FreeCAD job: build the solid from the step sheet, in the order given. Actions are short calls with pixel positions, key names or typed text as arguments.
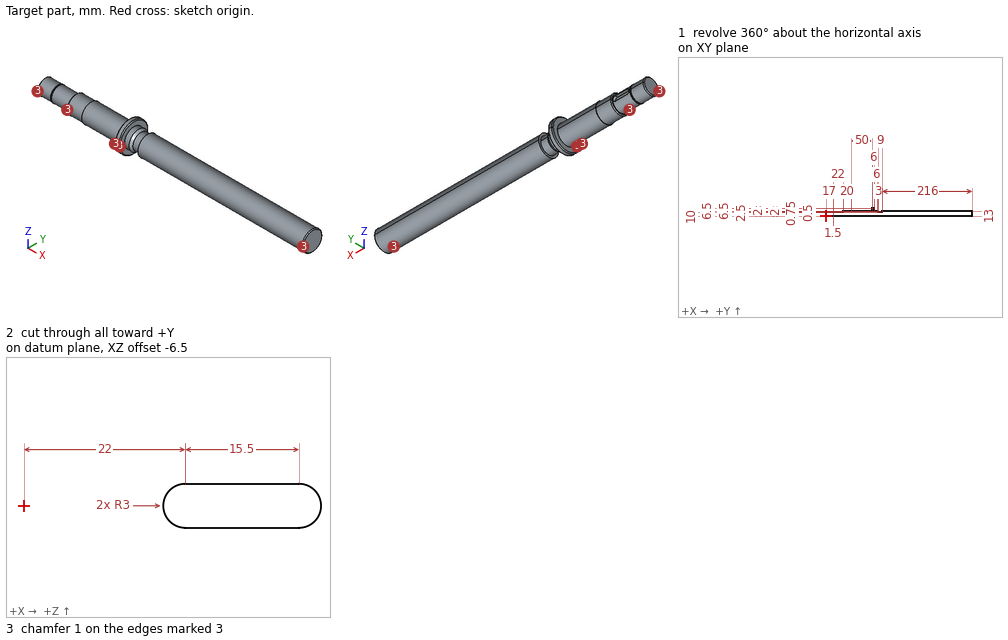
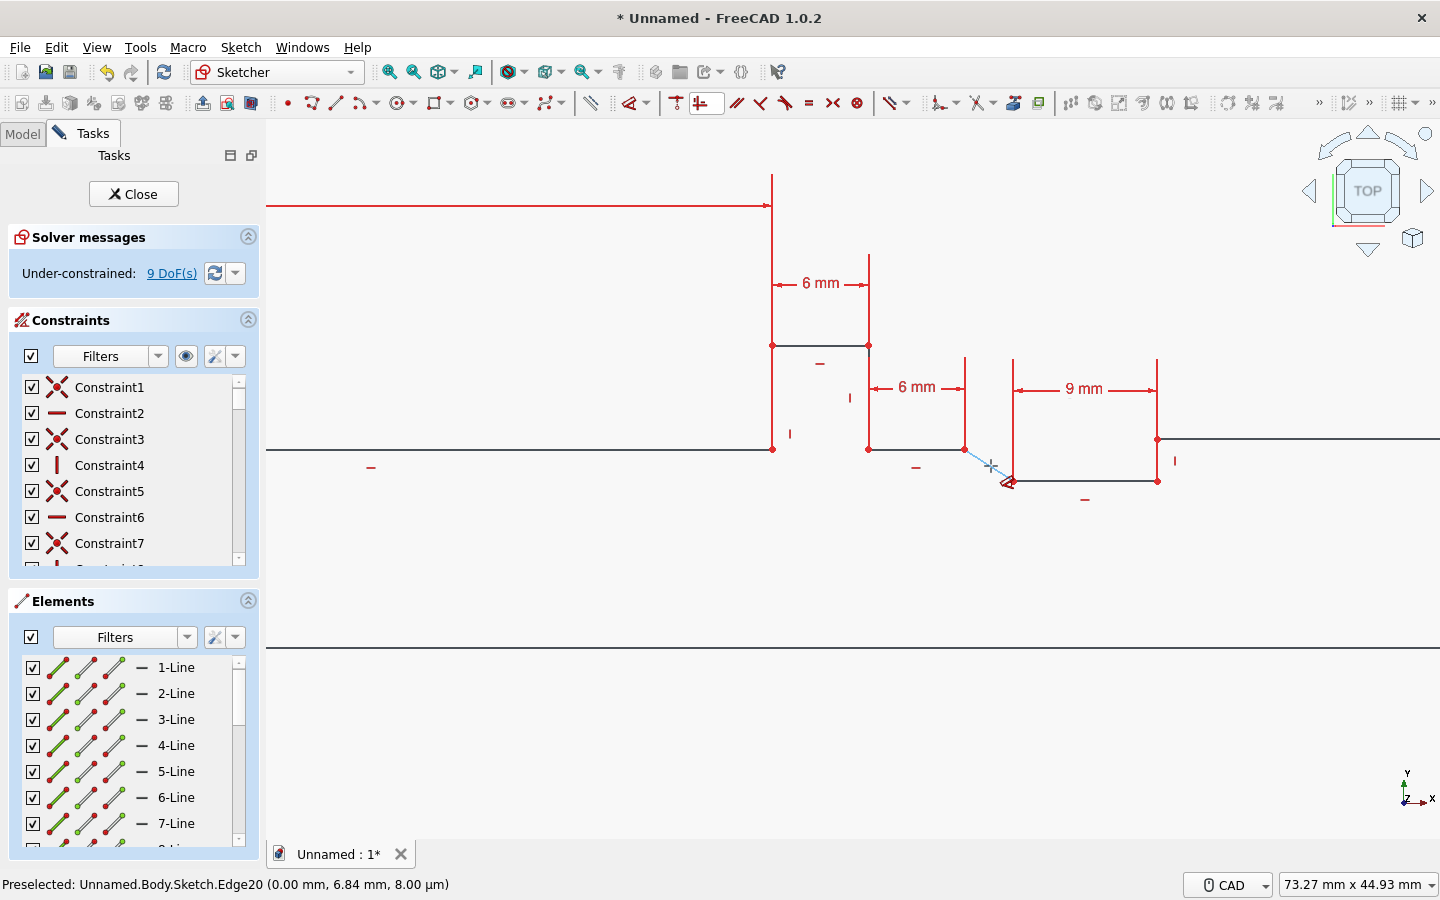
click(989, 465)
click(989, 416)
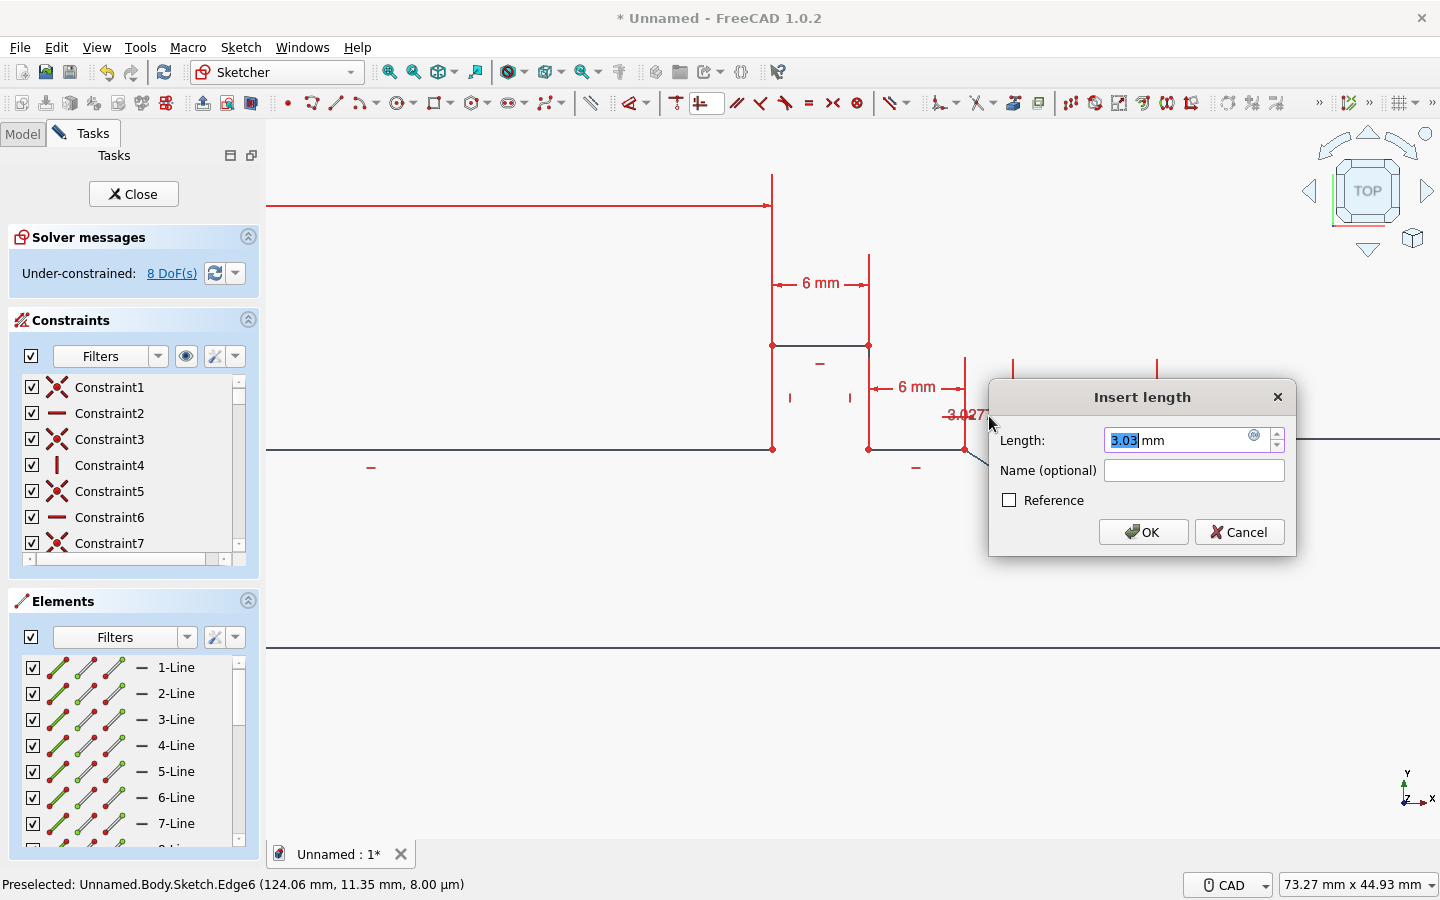
text(3)
key(Return)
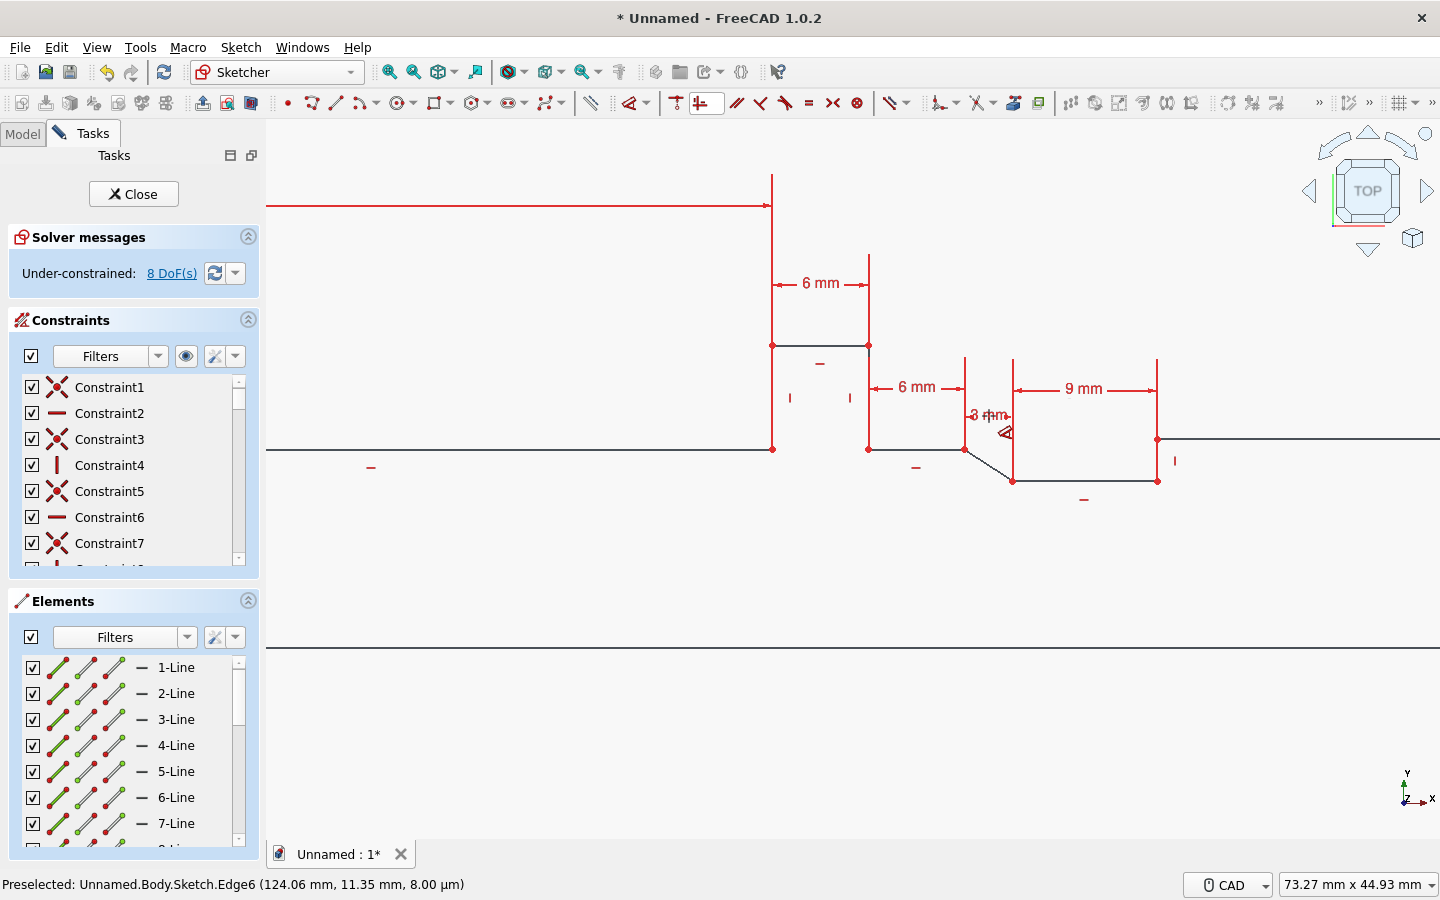
scroll(998, 472, up, 2)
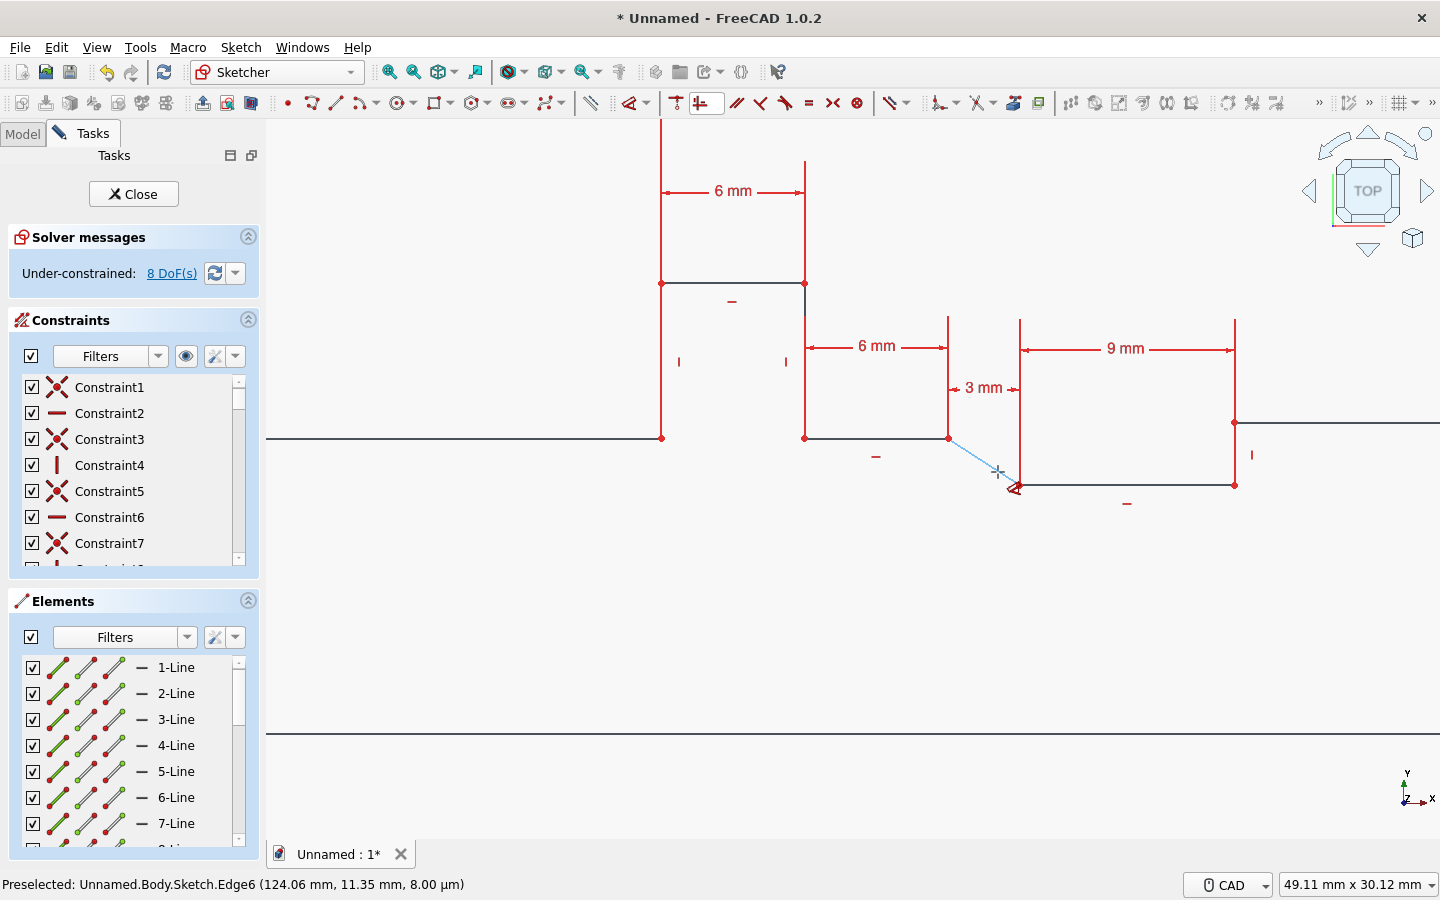
click(998, 471)
click(914, 462)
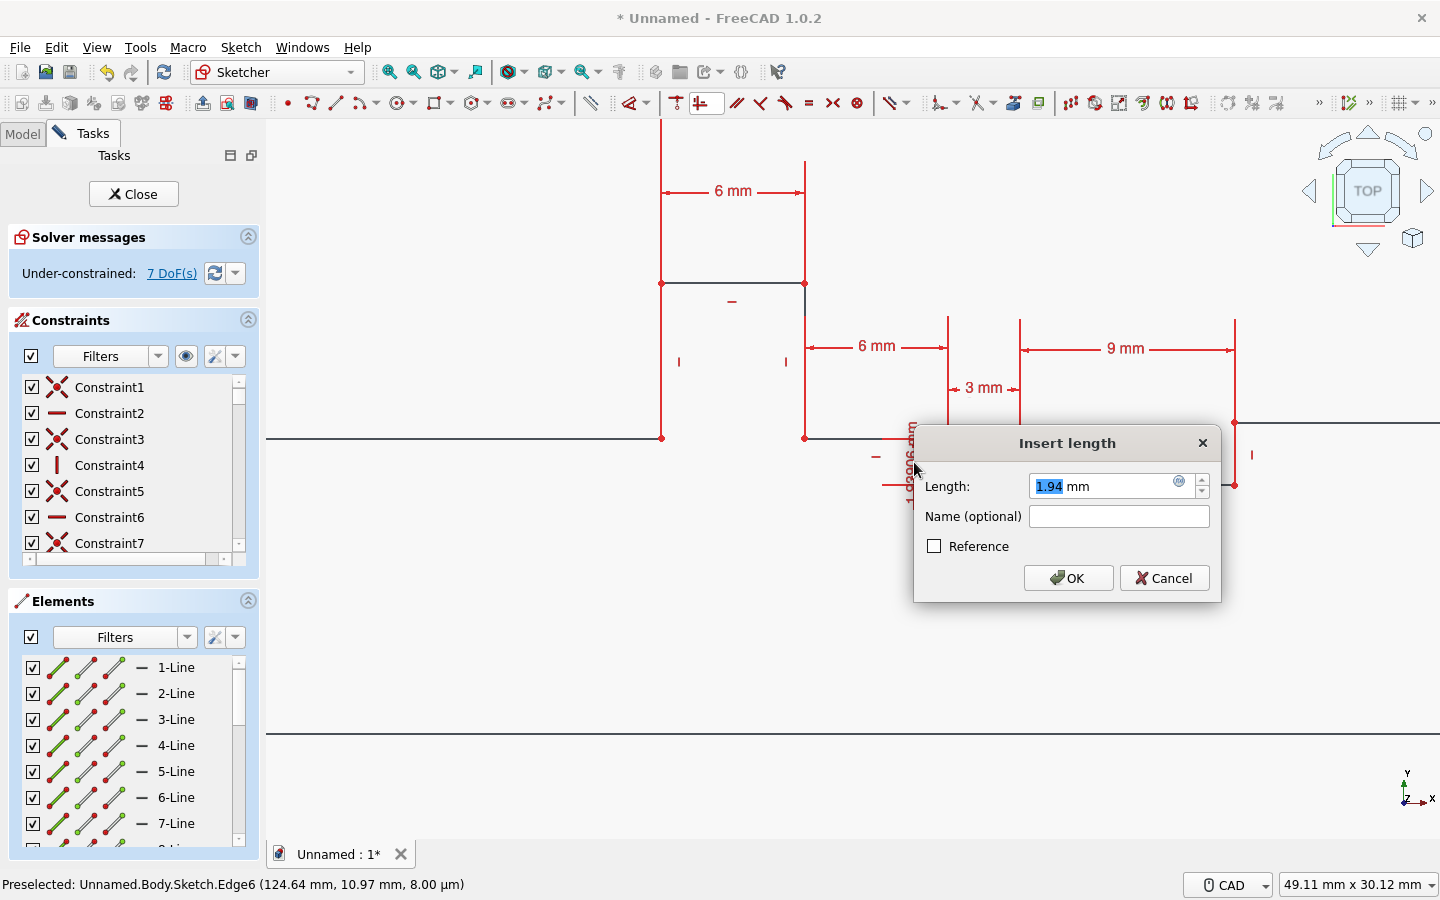
text(2)
key(Return)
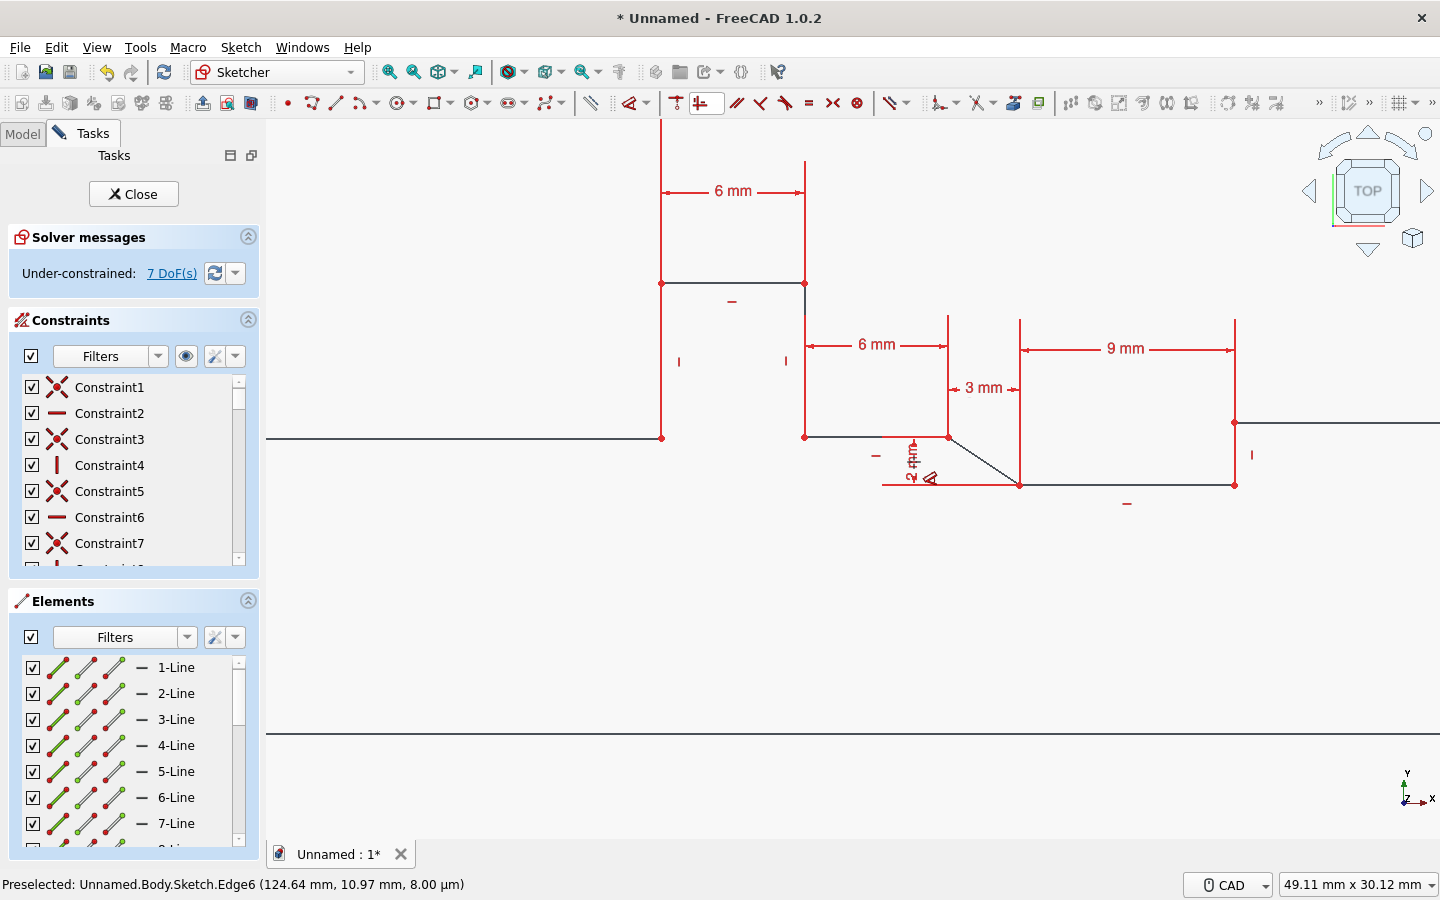
scroll(642, 476, down, 12)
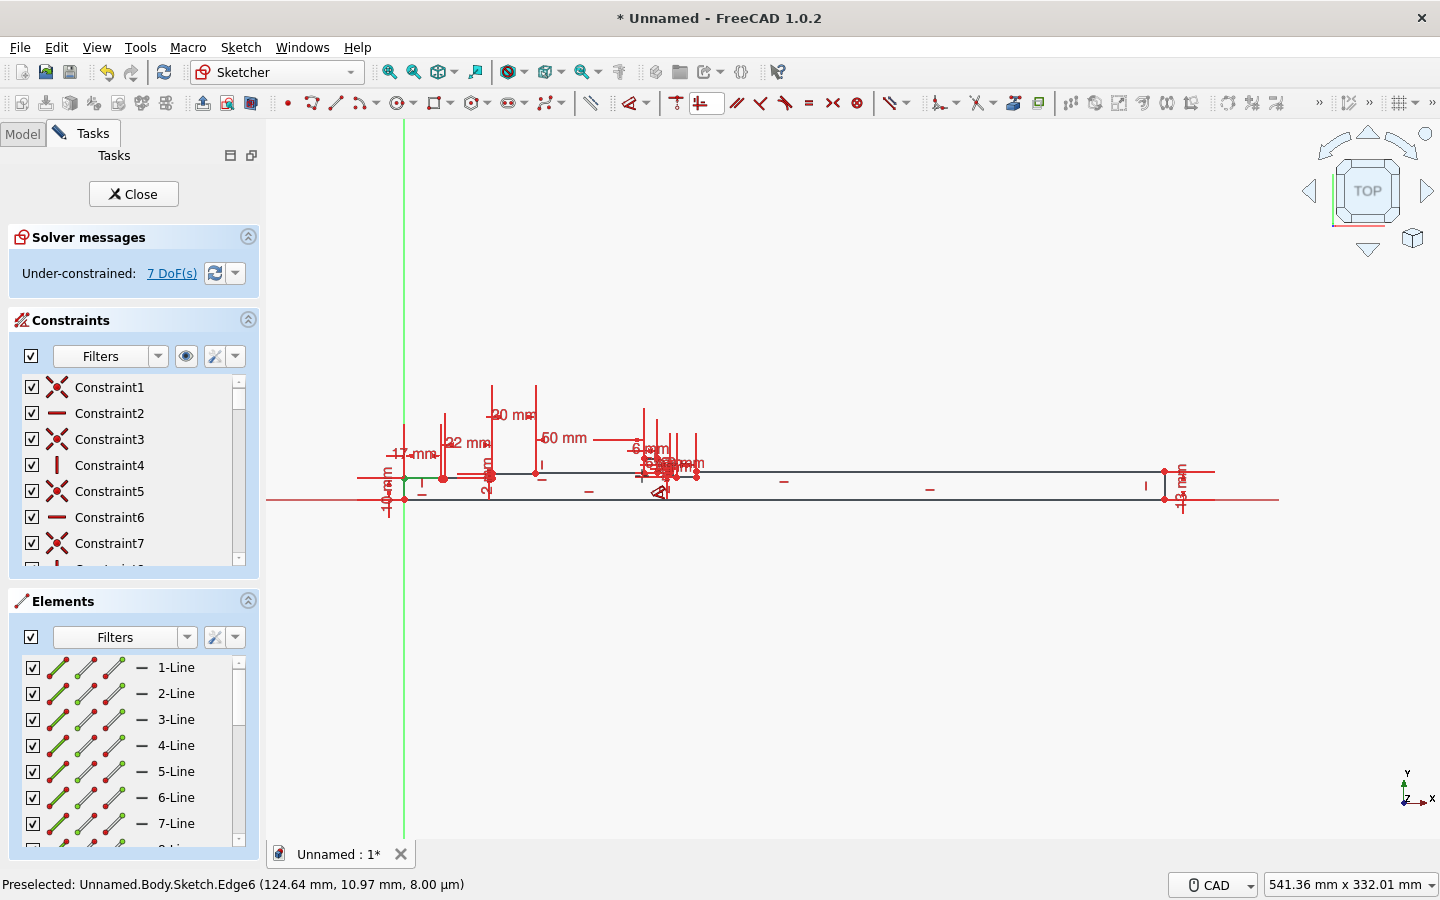
click(1024, 472)
click(930, 438)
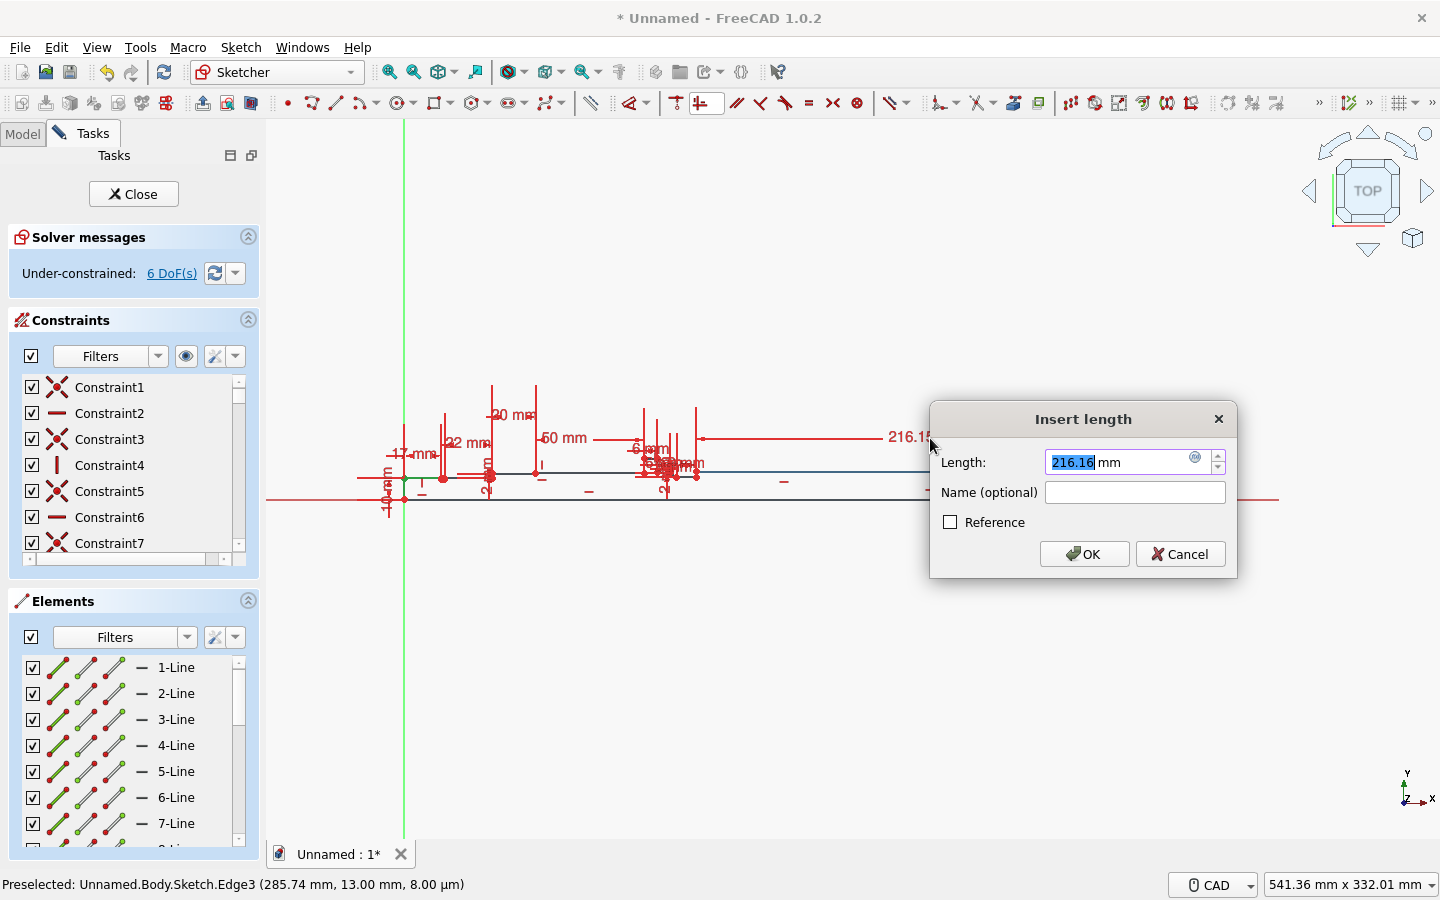
text(216)
key(Return)